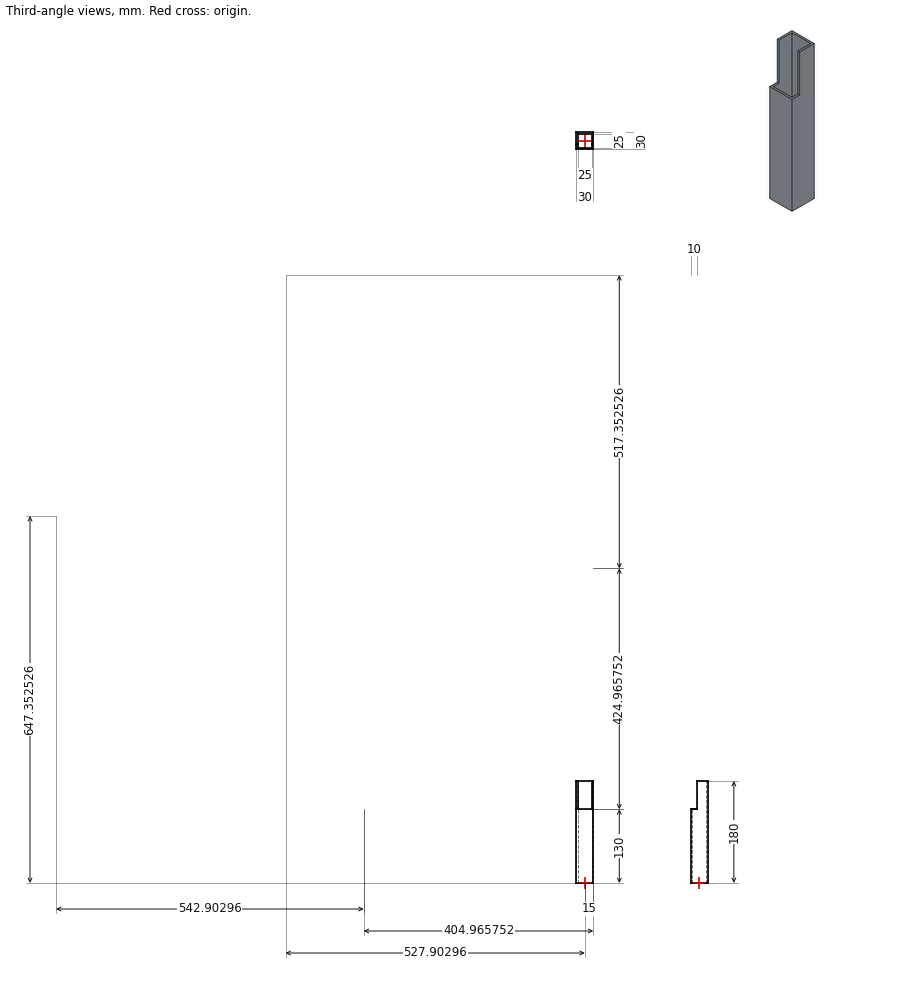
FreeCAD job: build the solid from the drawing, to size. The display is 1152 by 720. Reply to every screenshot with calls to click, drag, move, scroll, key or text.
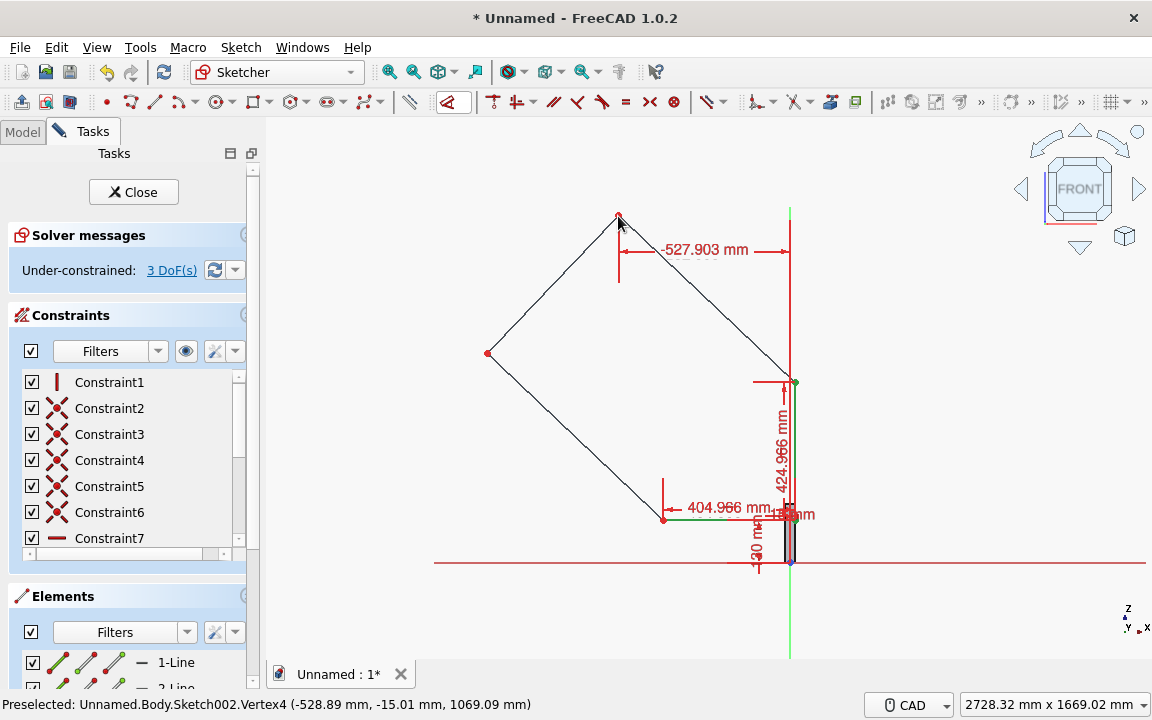
click(540, 404)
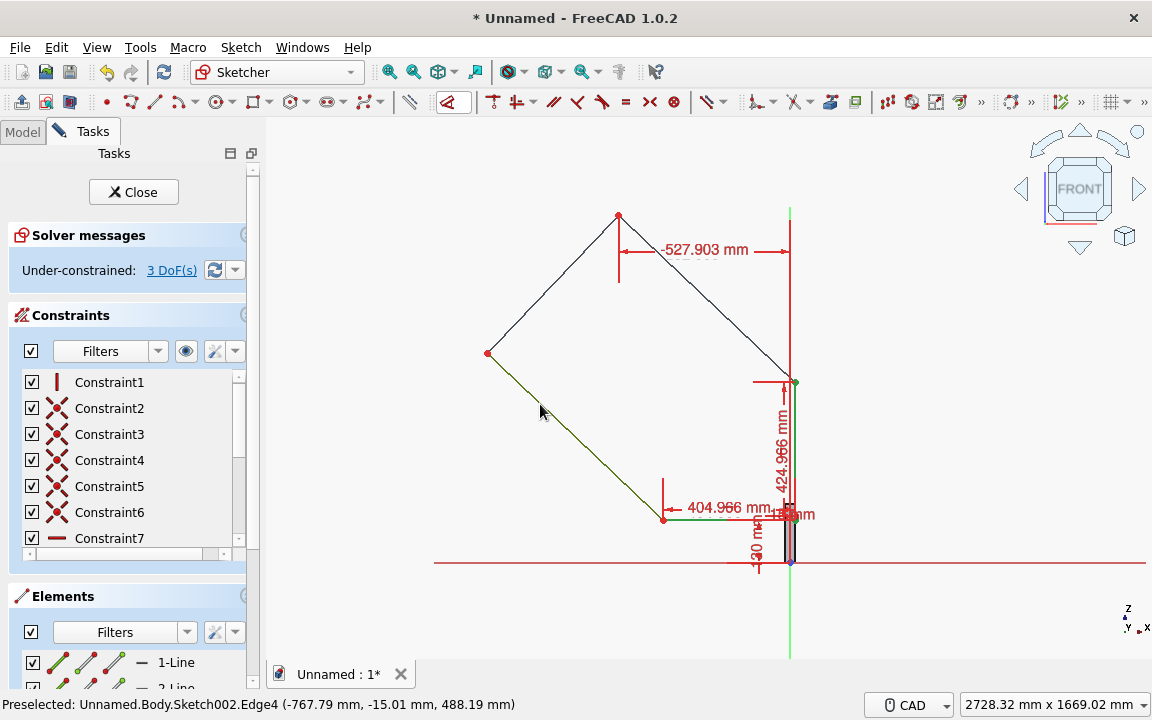
click(466, 102)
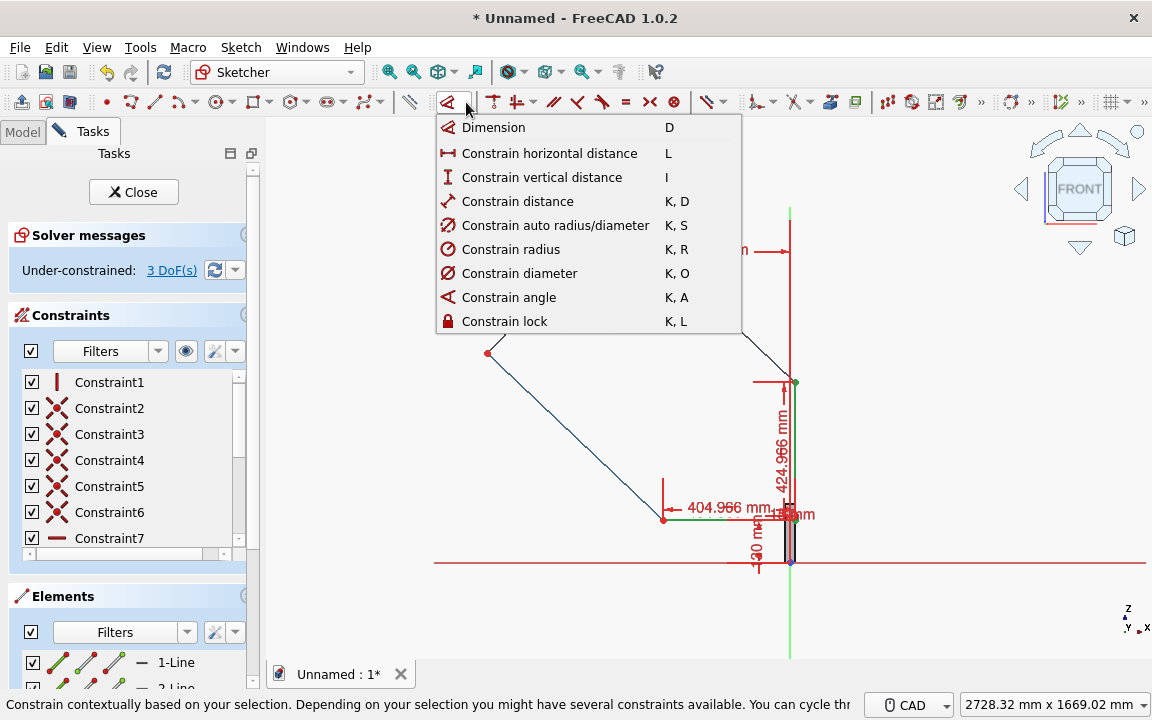
click(589, 153)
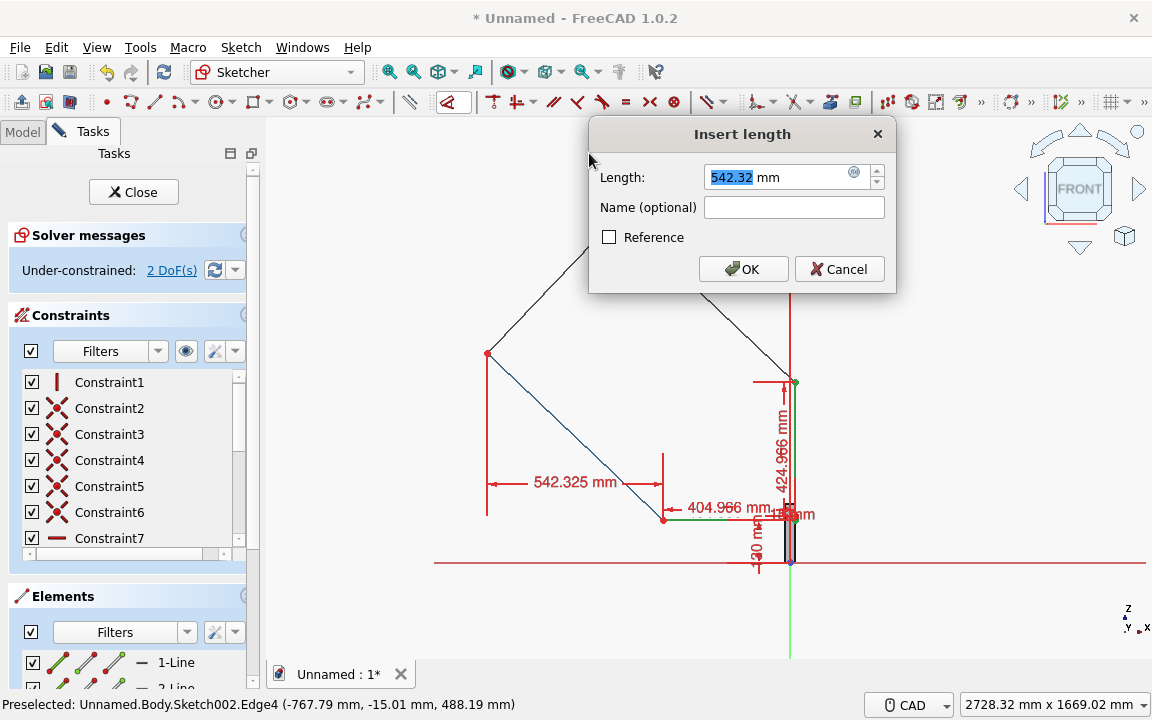
text(542.90296)
key(Return)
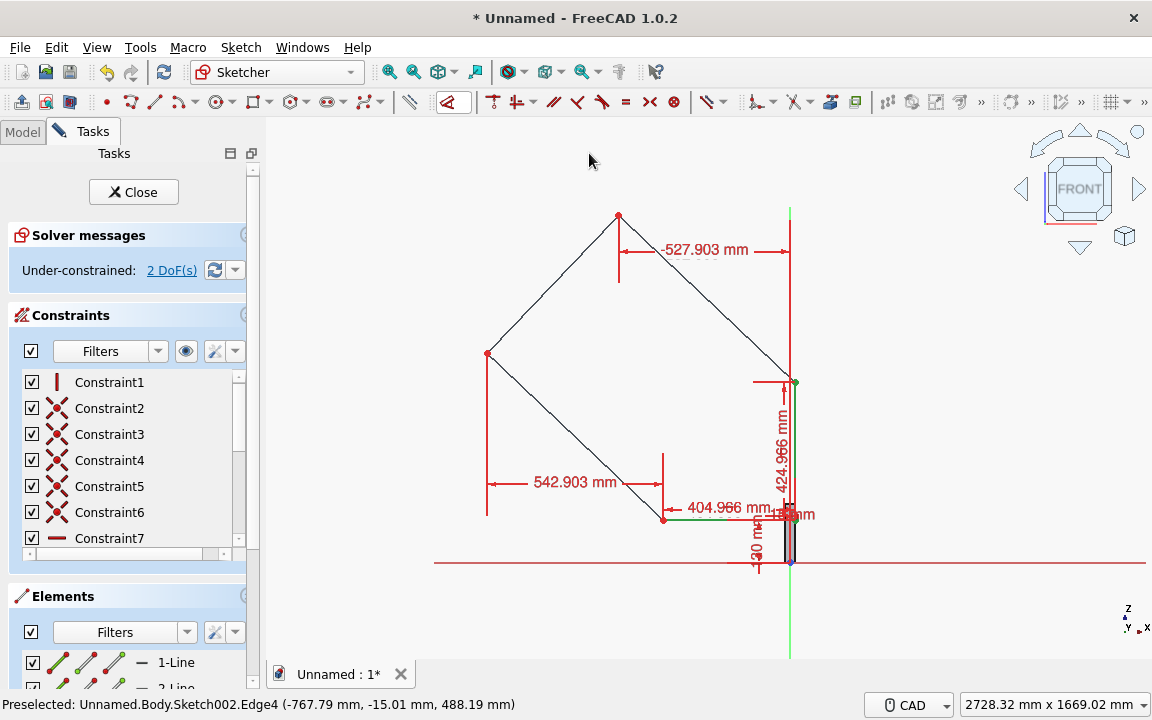
click(487, 354)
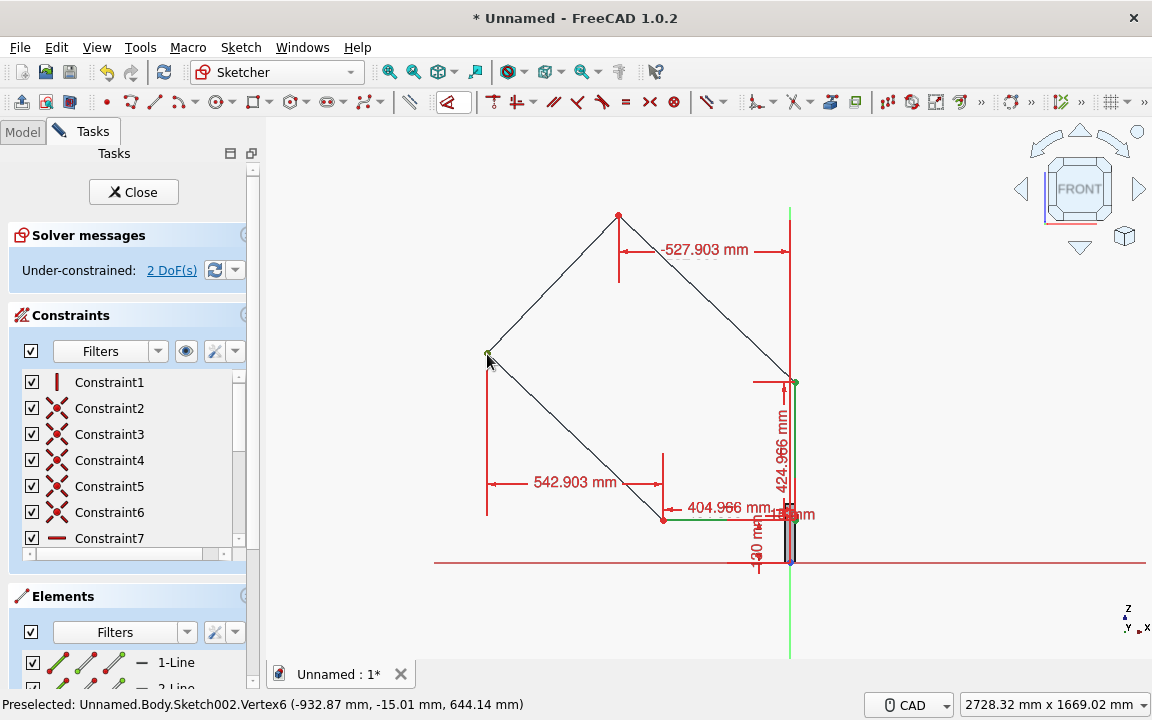
key(i)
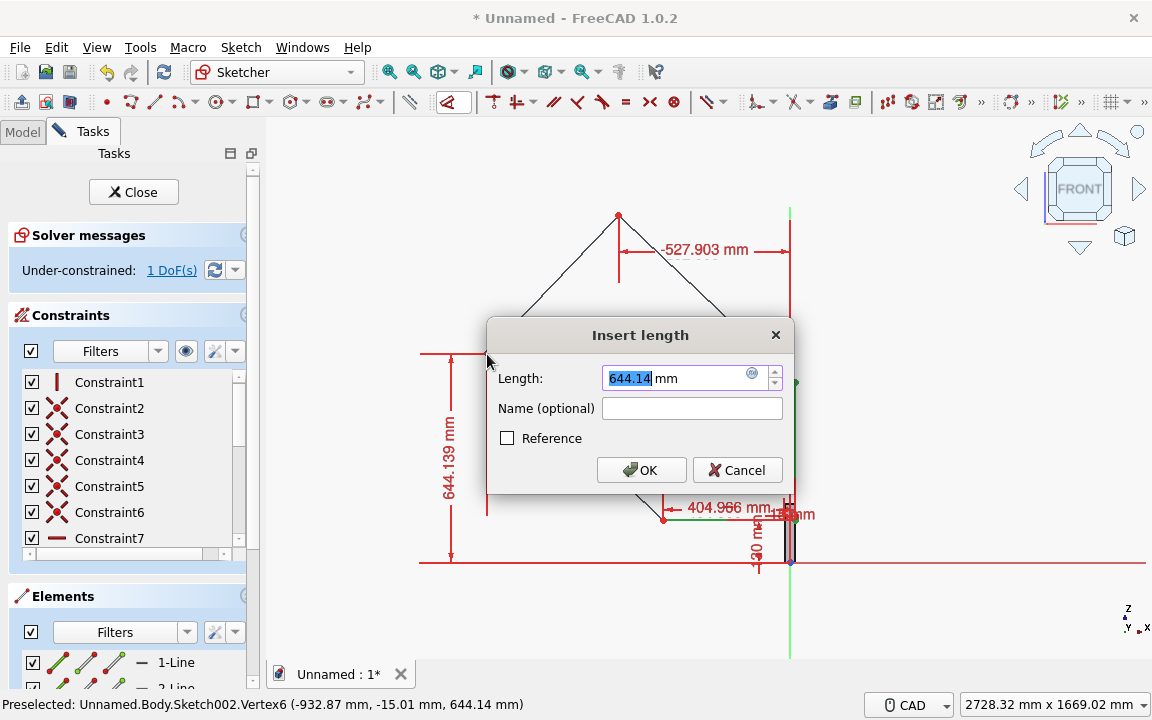
text(647.352526)
key(Return)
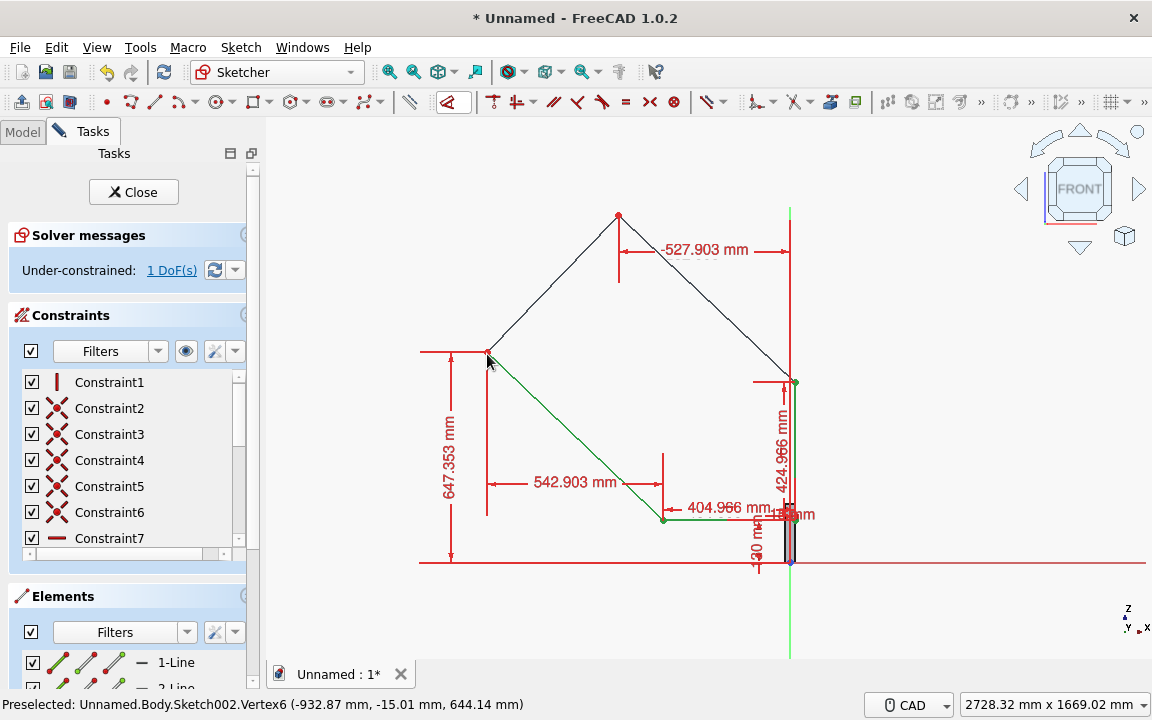
click(742, 332)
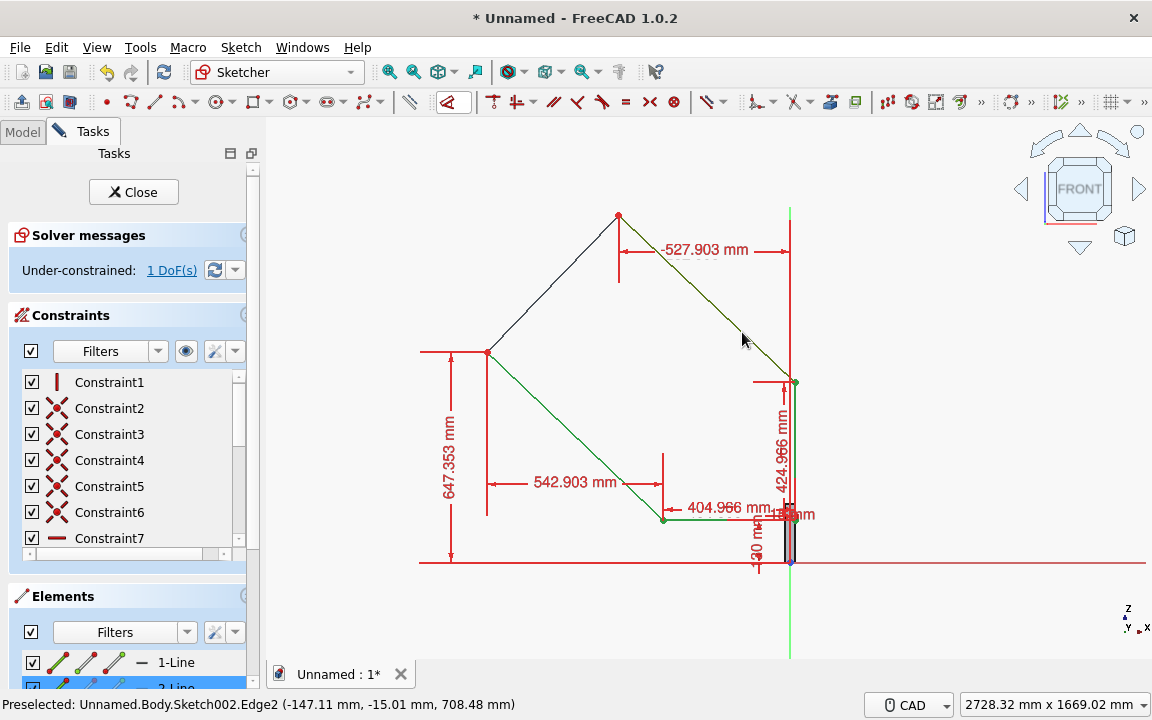
key(i)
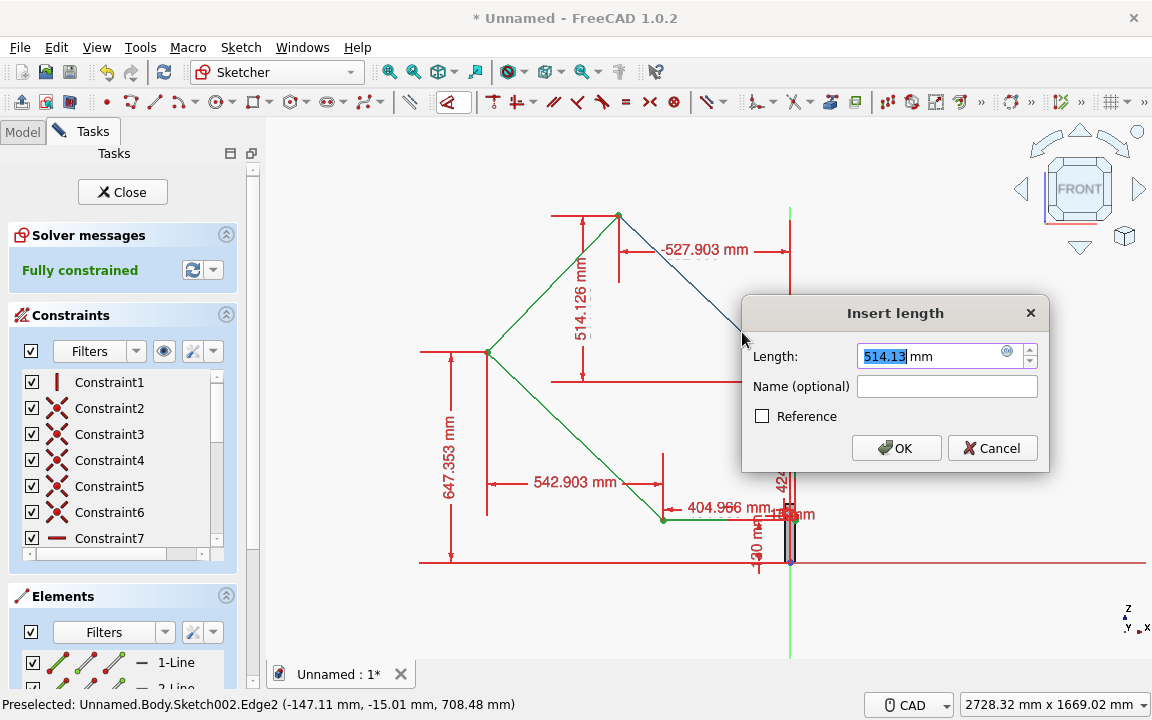
text(517.352526)
key(Return)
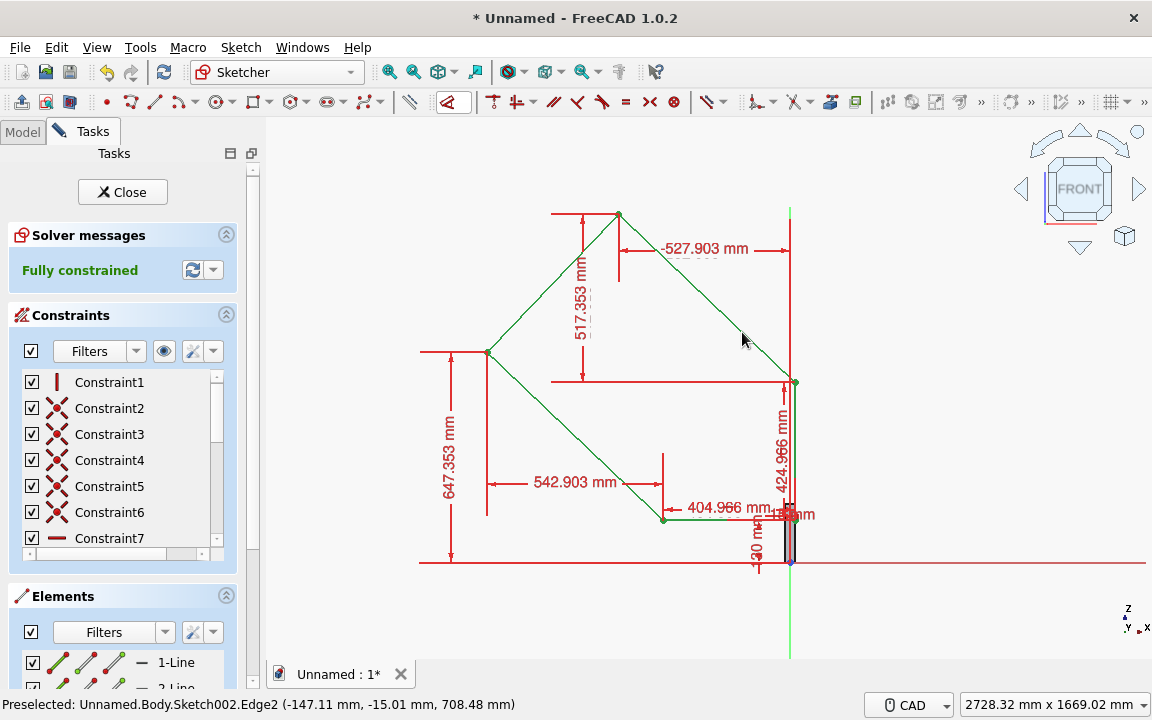
click(123, 192)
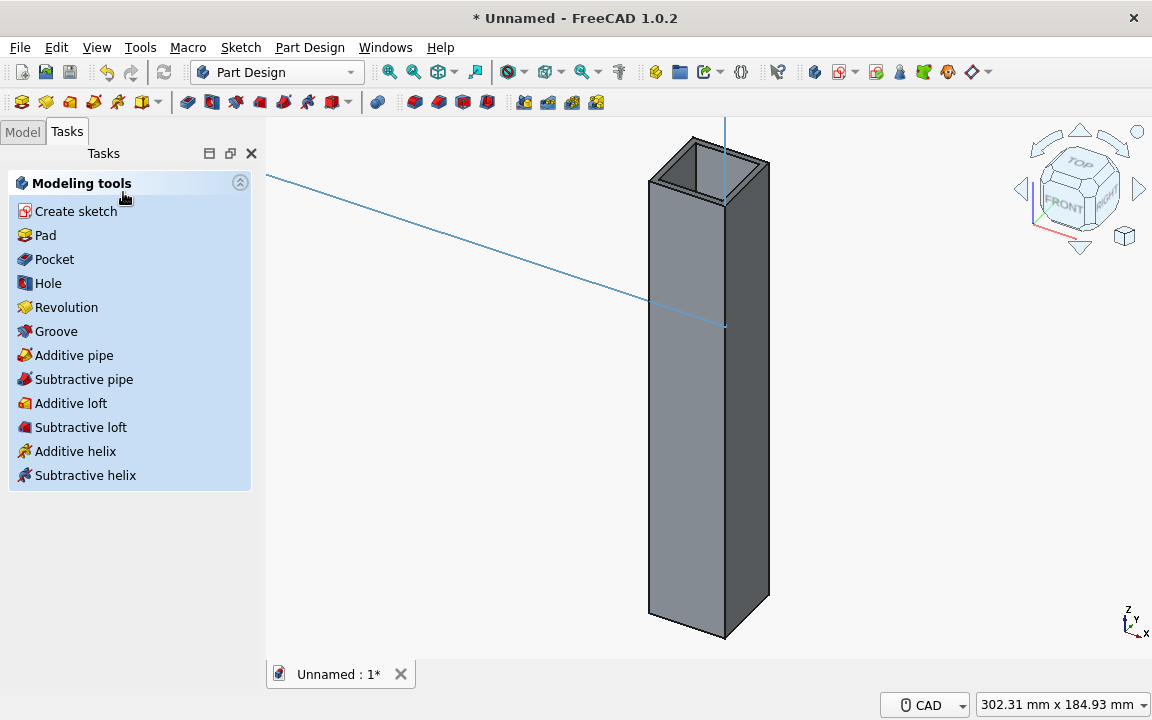
click(188, 102)